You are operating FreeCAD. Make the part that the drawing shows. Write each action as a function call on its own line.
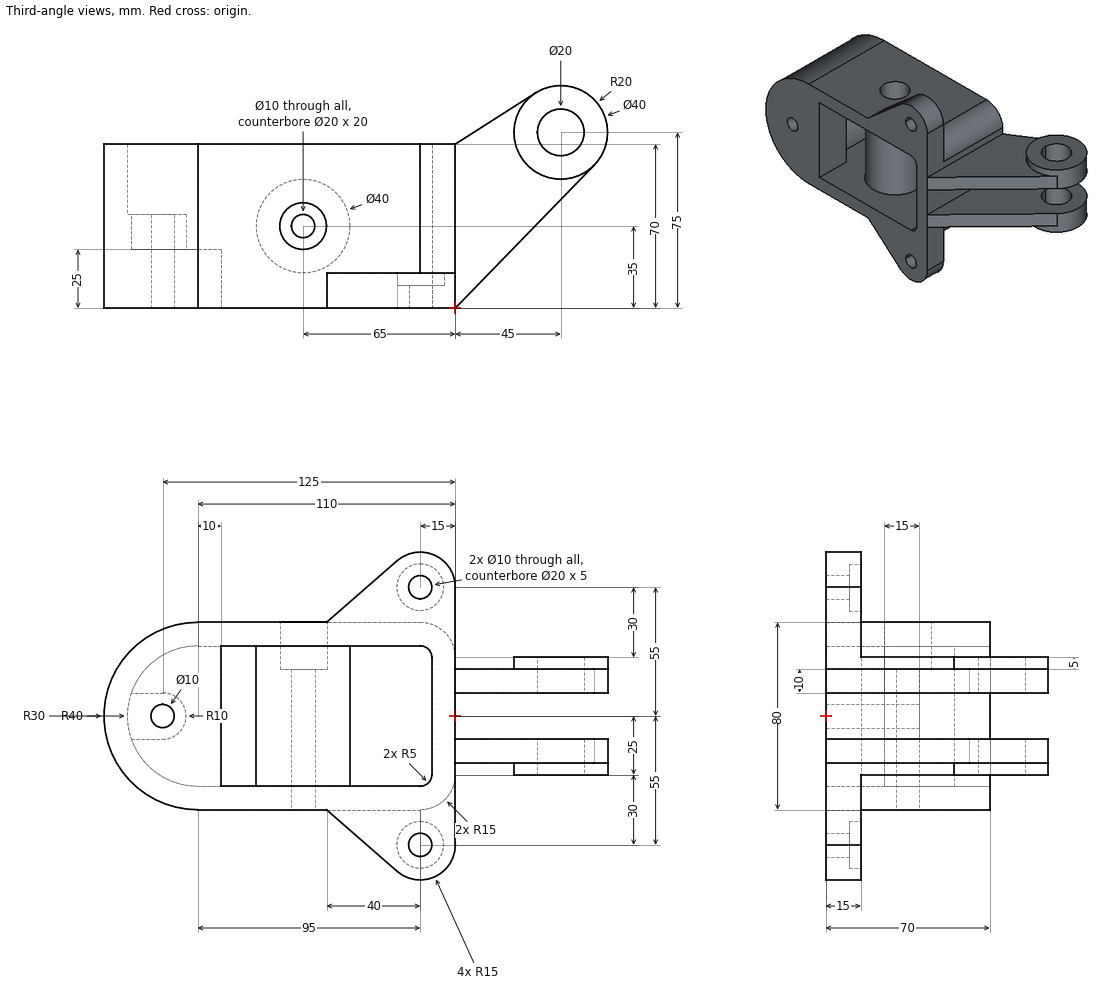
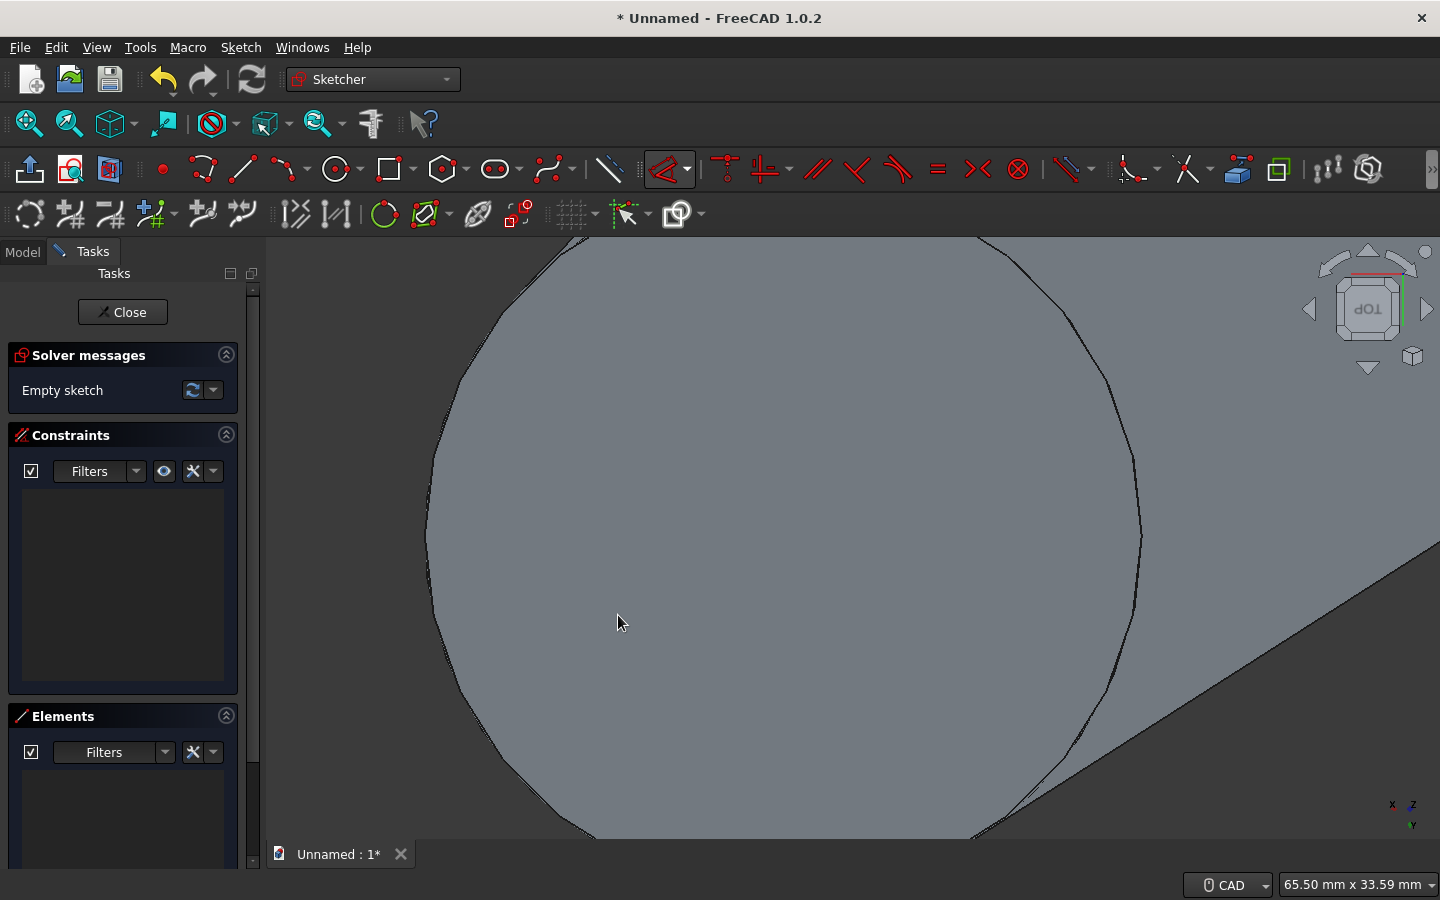
key(g)
key(c)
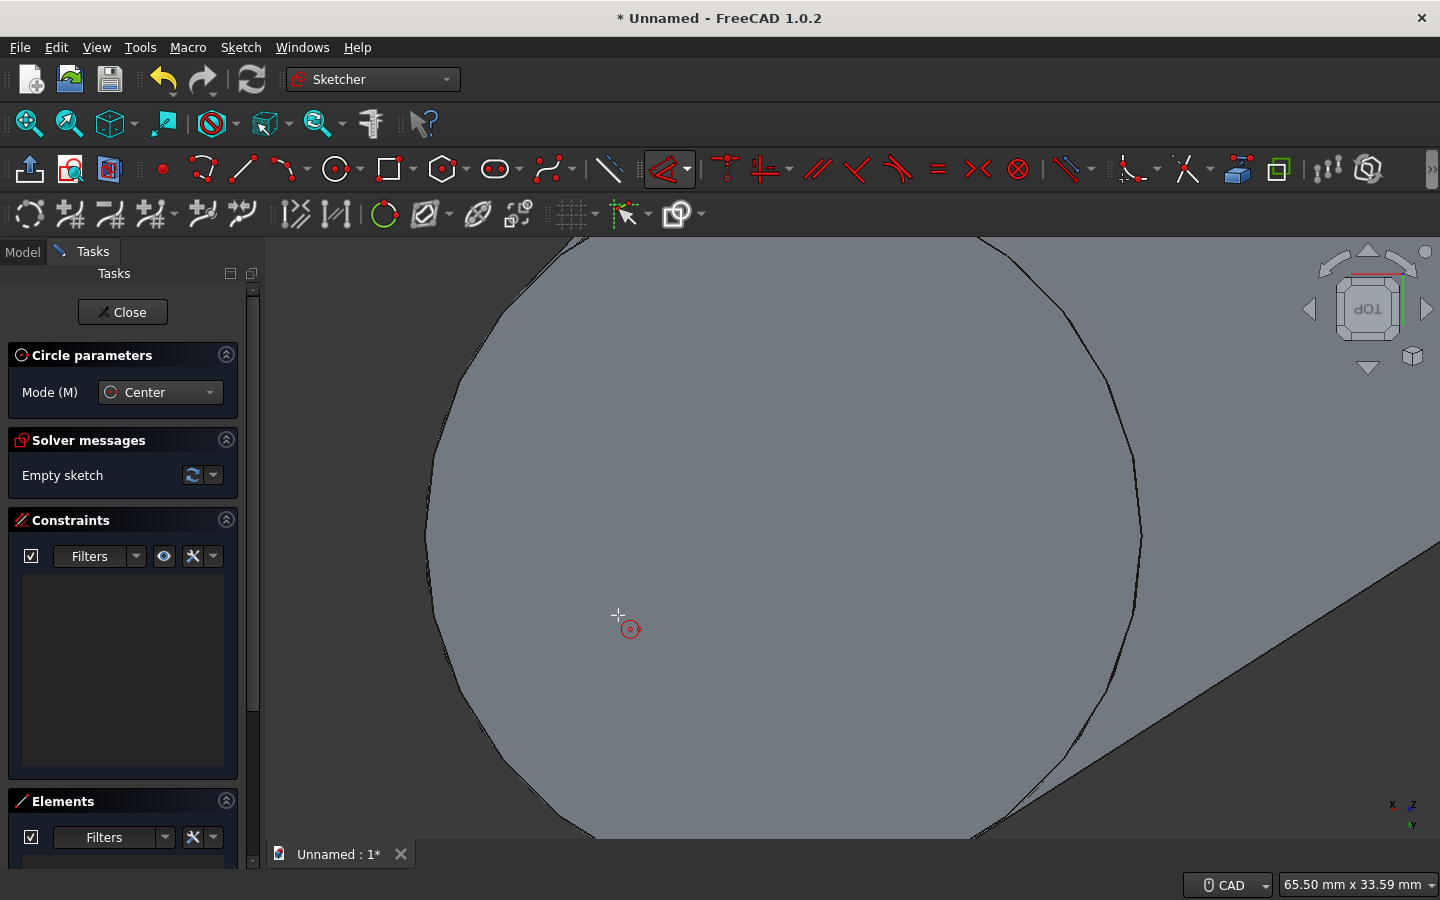
click(783, 536)
move(910, 409)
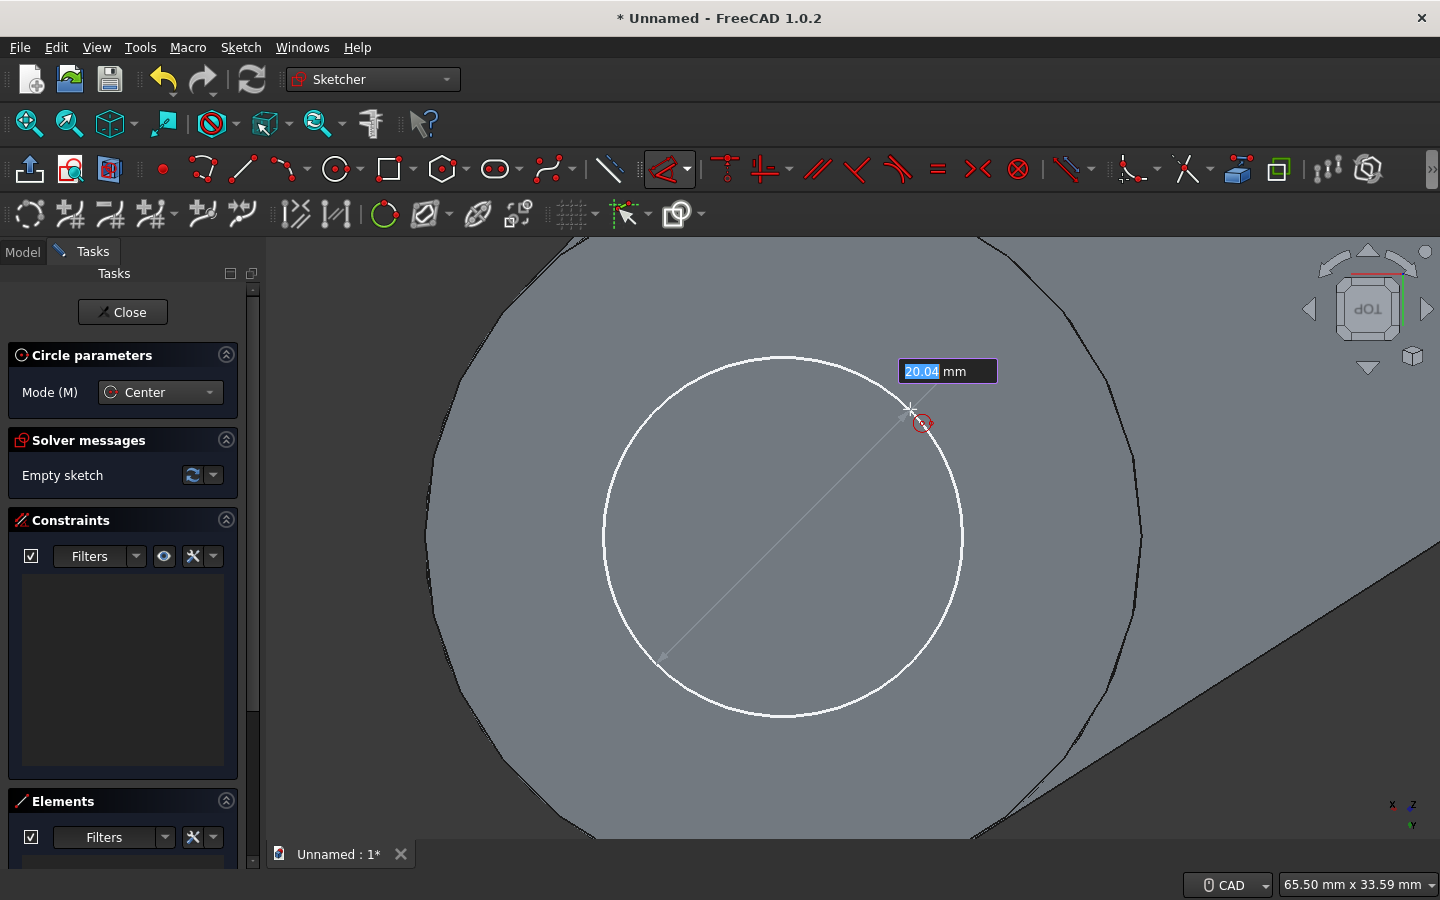
text(20)
key(Return)
key(Escape)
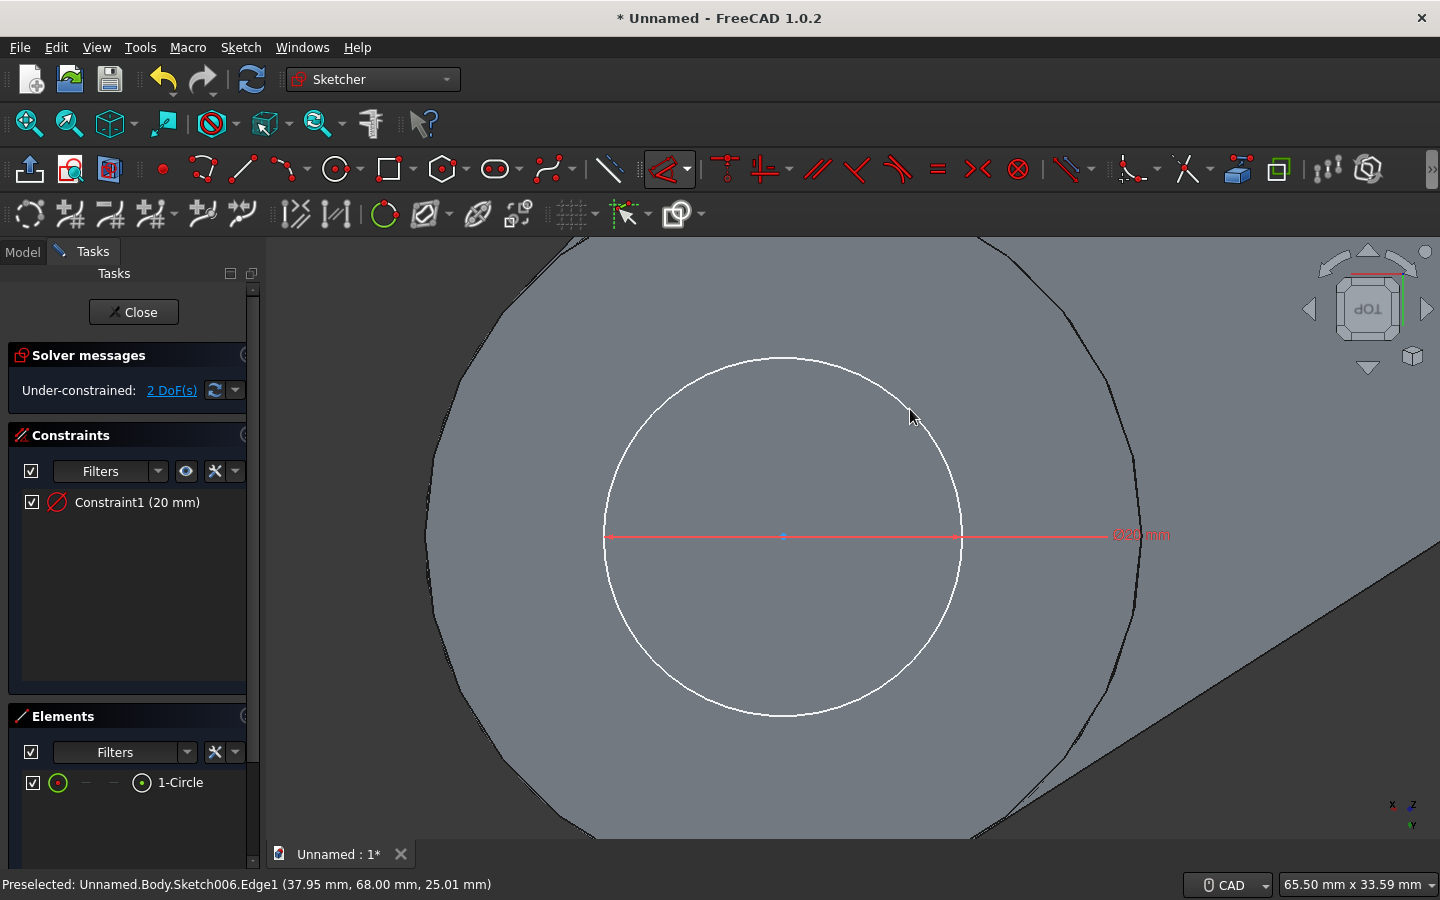
click(783, 537)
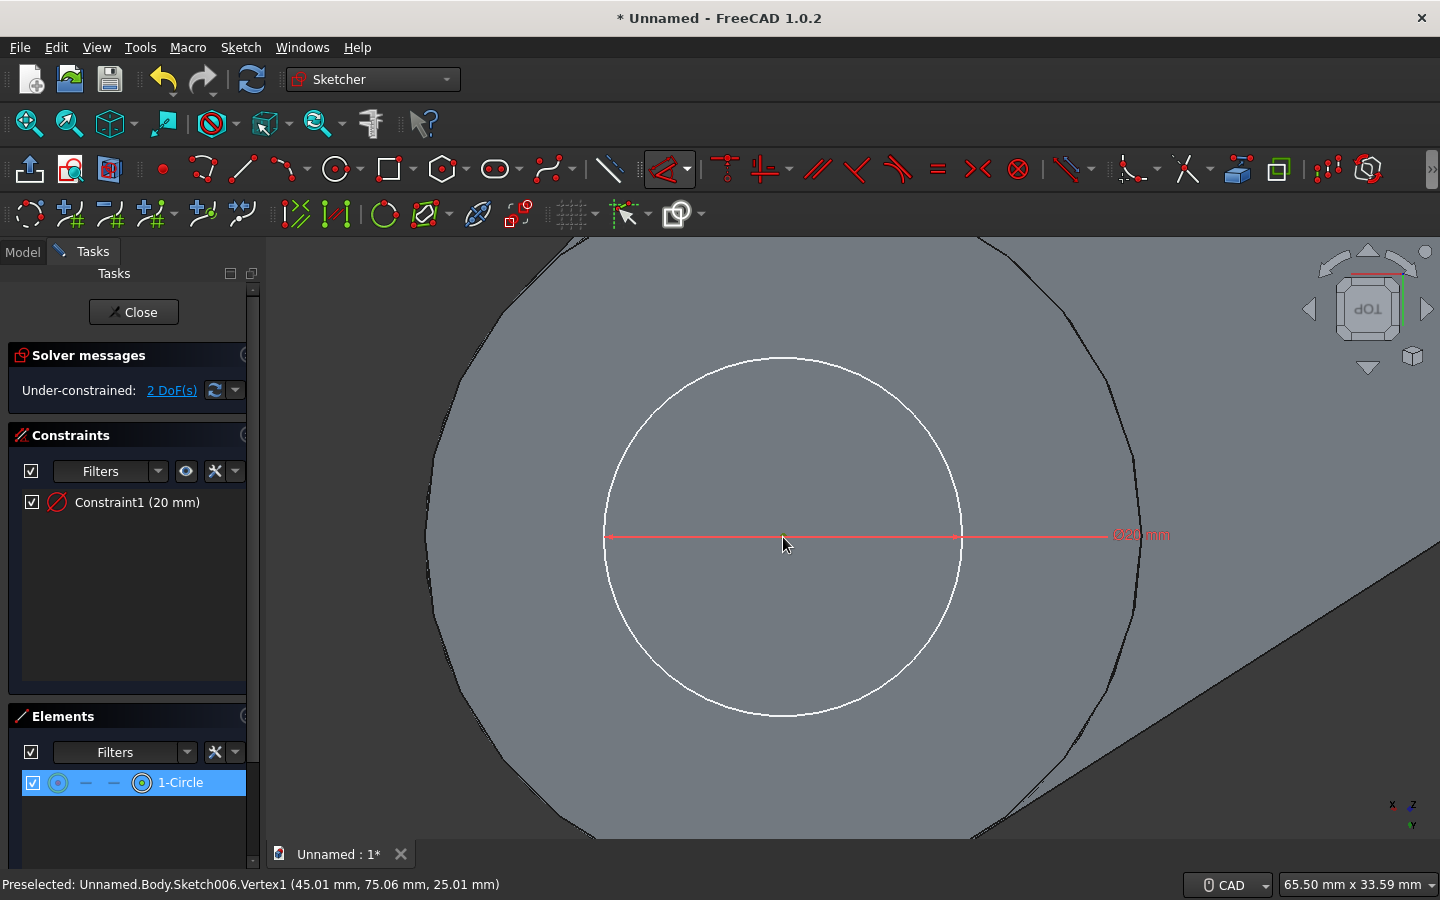
key(l)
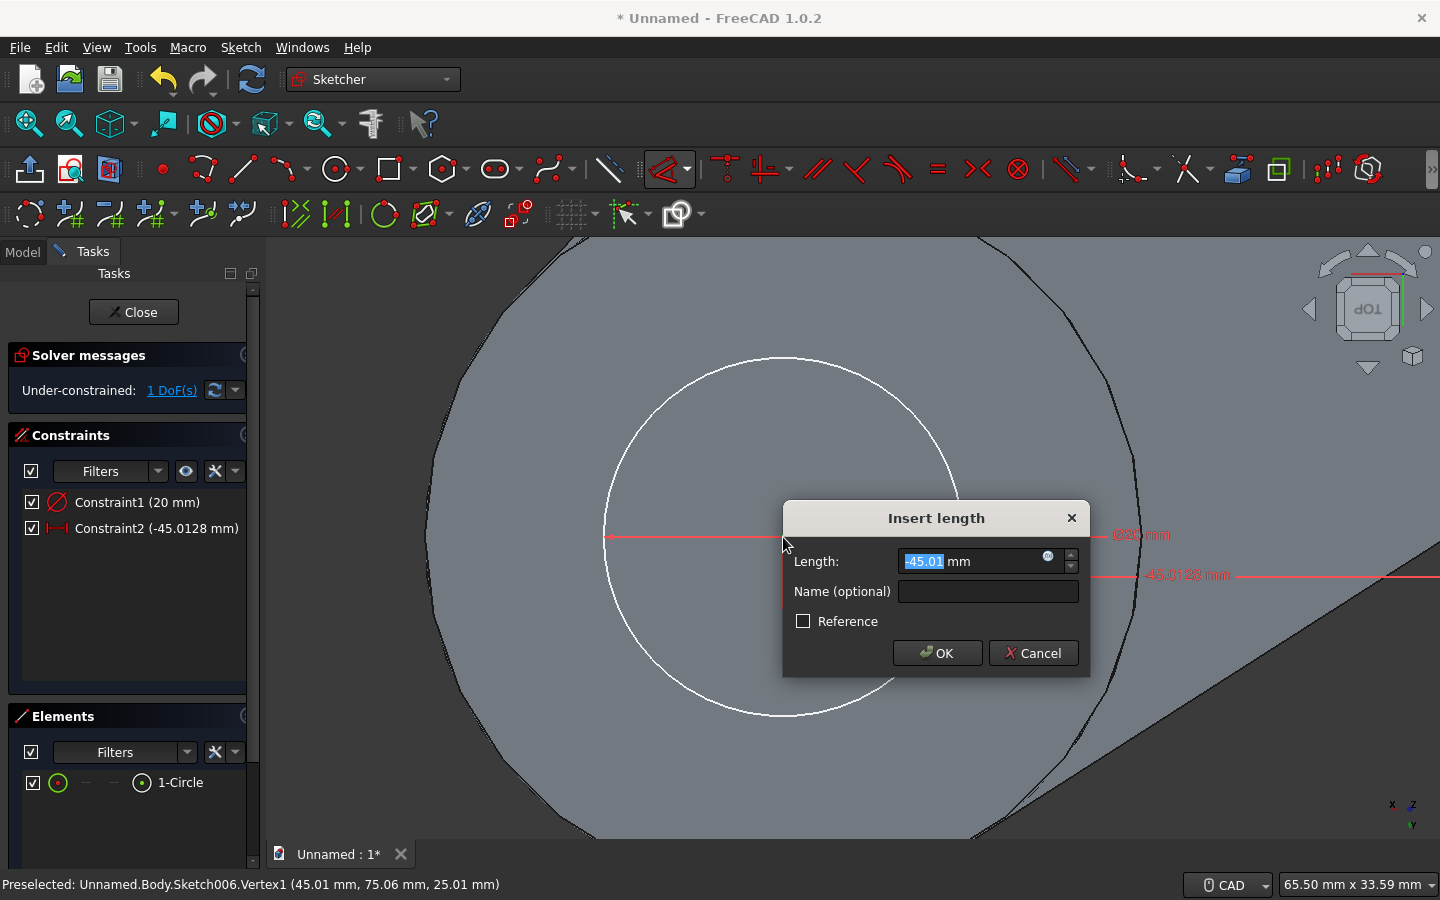
text(-45)
key(Return)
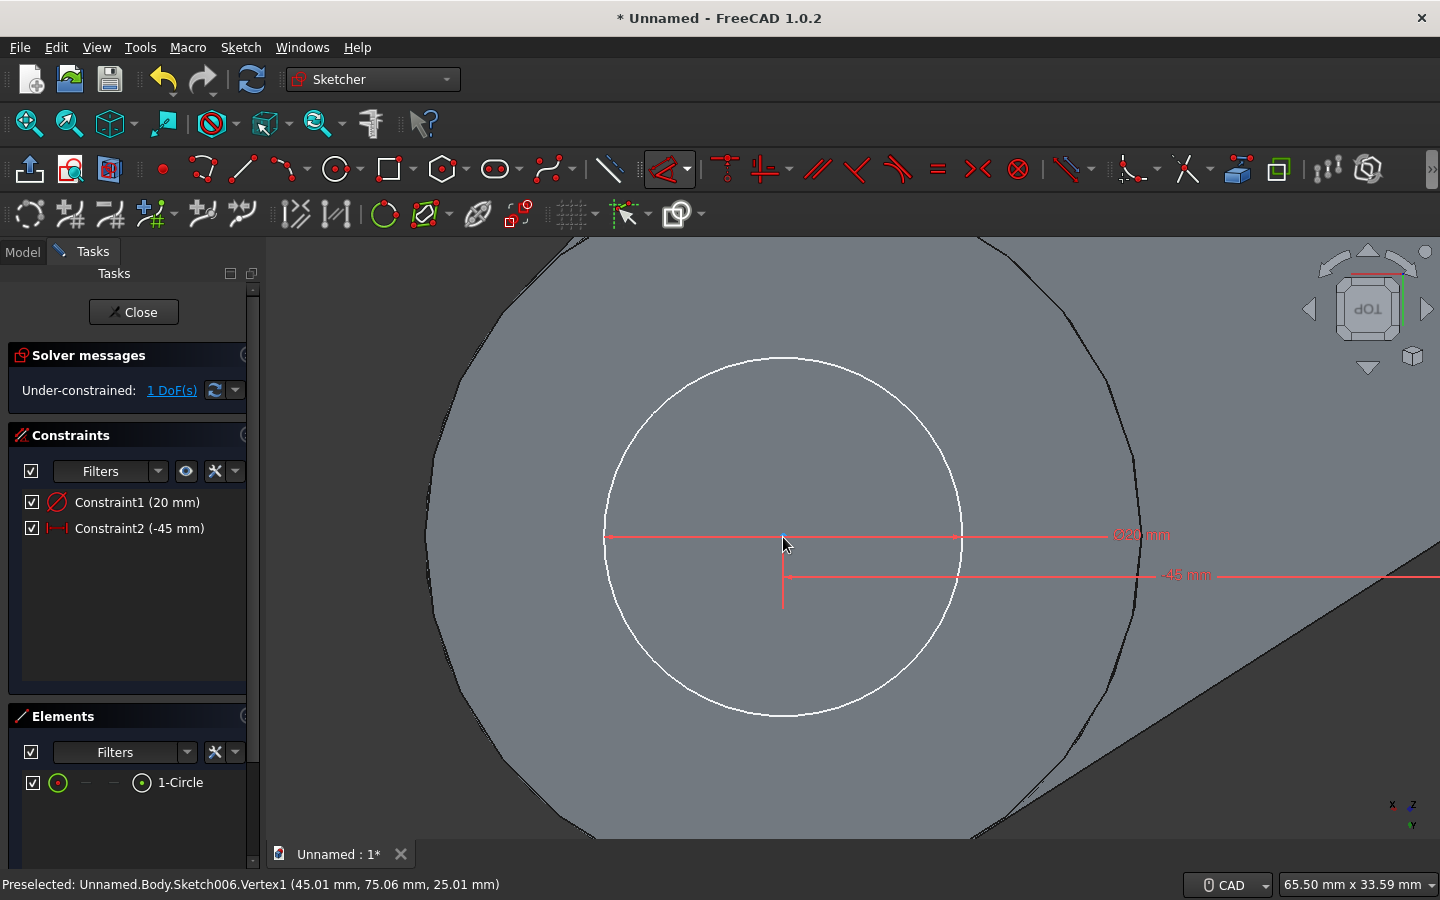
click(783, 537)